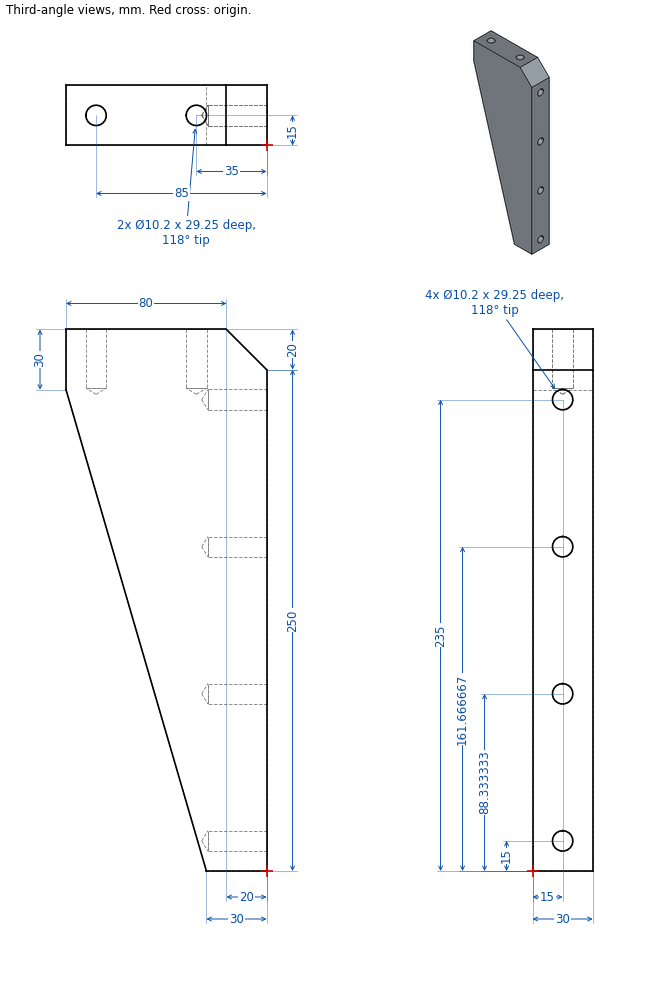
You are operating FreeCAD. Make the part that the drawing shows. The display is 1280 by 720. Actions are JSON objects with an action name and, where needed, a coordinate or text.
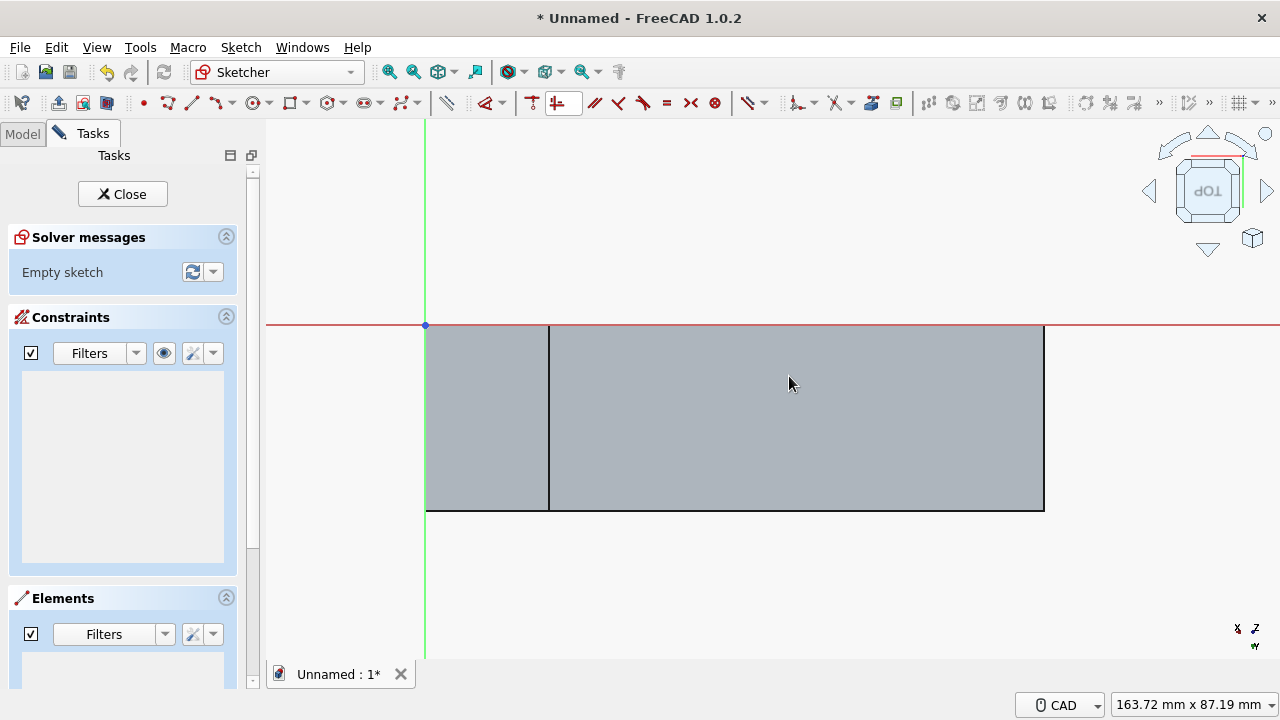
{"action": "key", "text": "g c"}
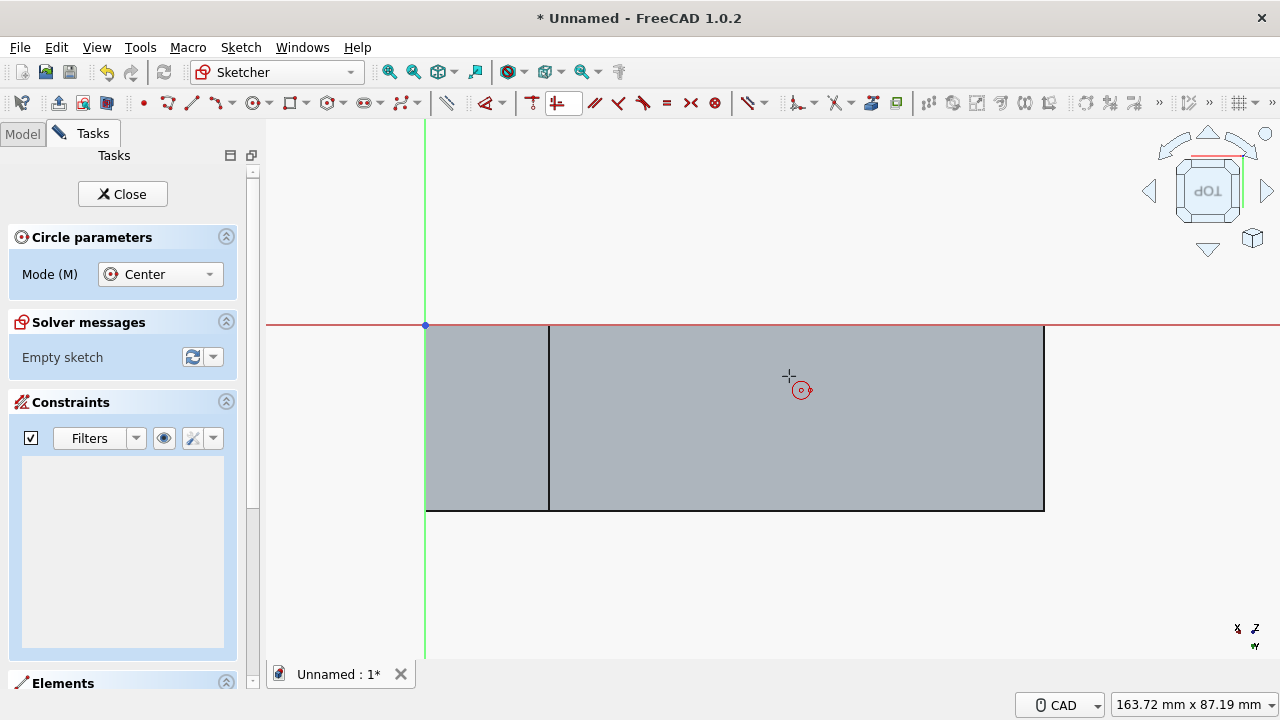
{"action": "left_click", "coordinate": [642, 418]}
{"action": "left_click", "coordinate": [664, 396]}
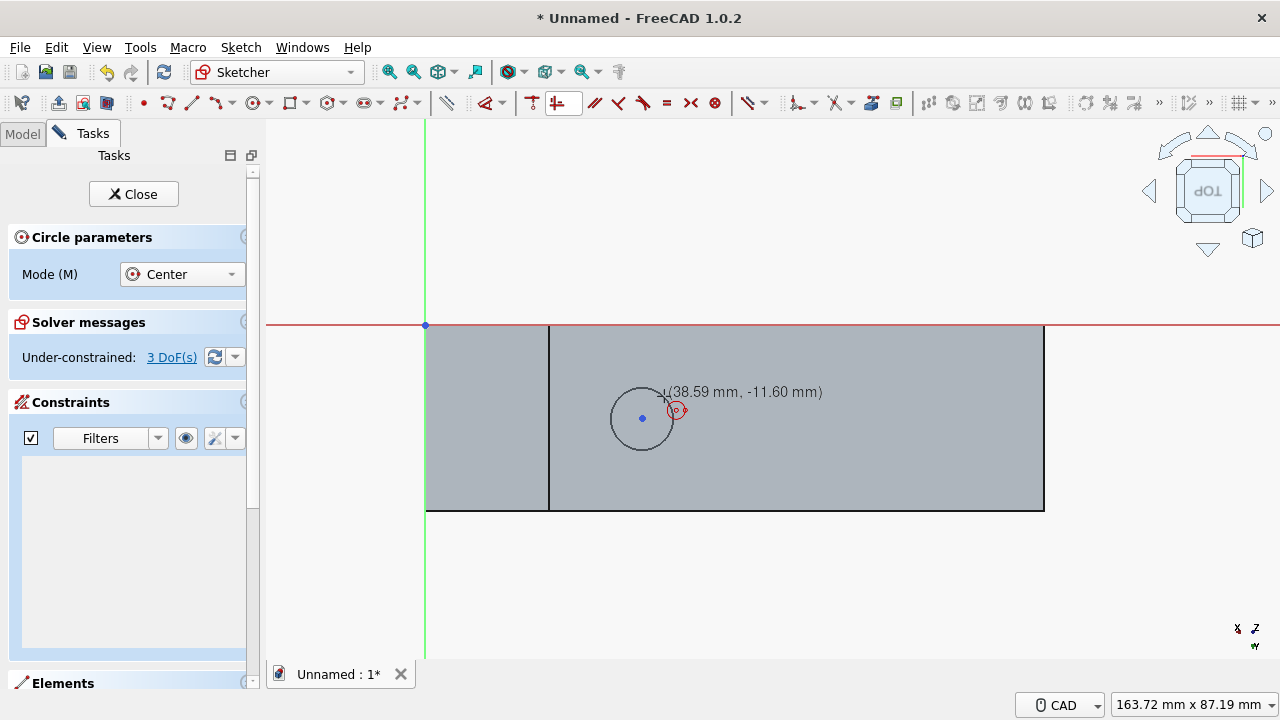
{"action": "left_click", "coordinate": [951, 418]}
{"action": "left_click", "coordinate": [974, 396]}
{"action": "key", "text": "Escape"}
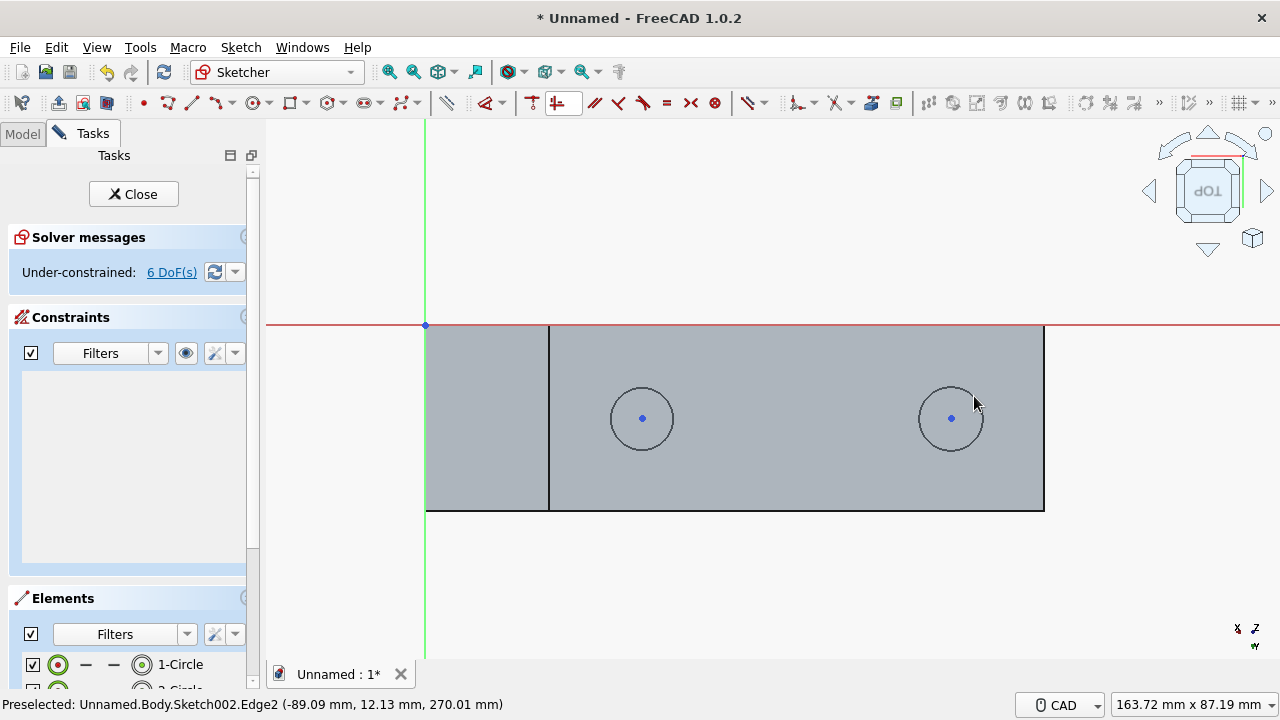
{"action": "left_click", "coordinate": [664, 397]}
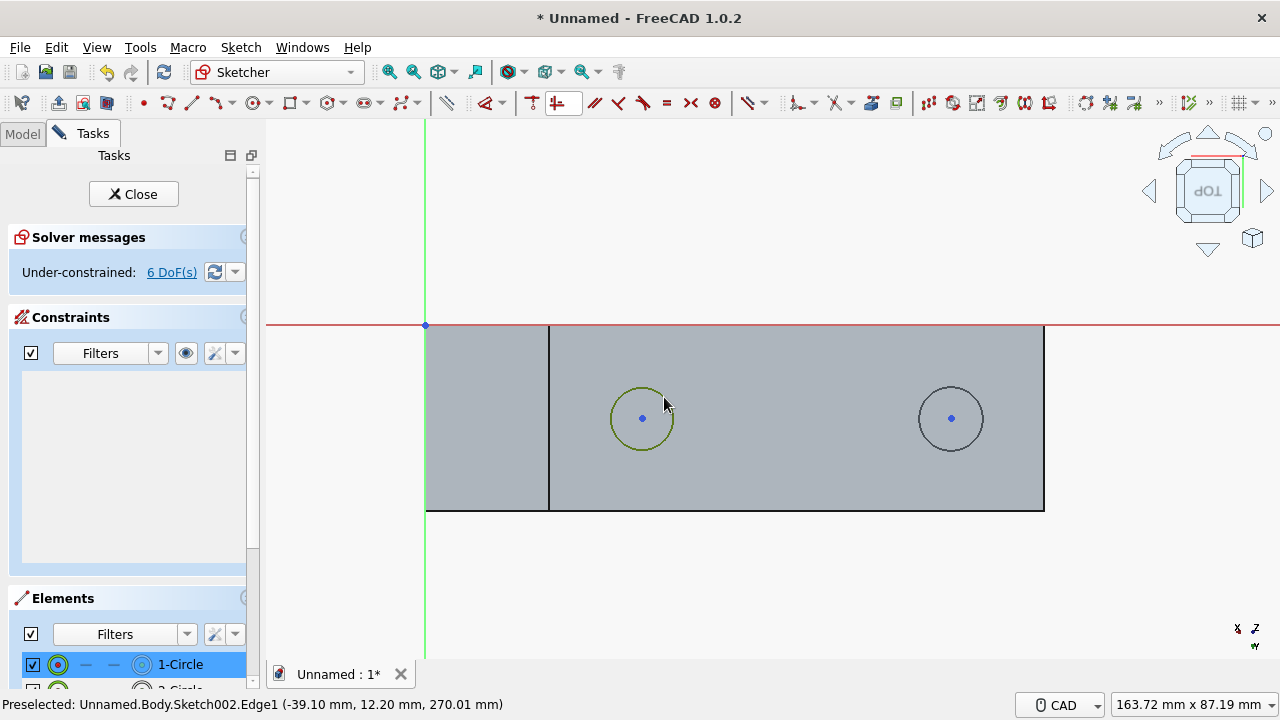
{"action": "left_click", "coordinate": [973, 396]}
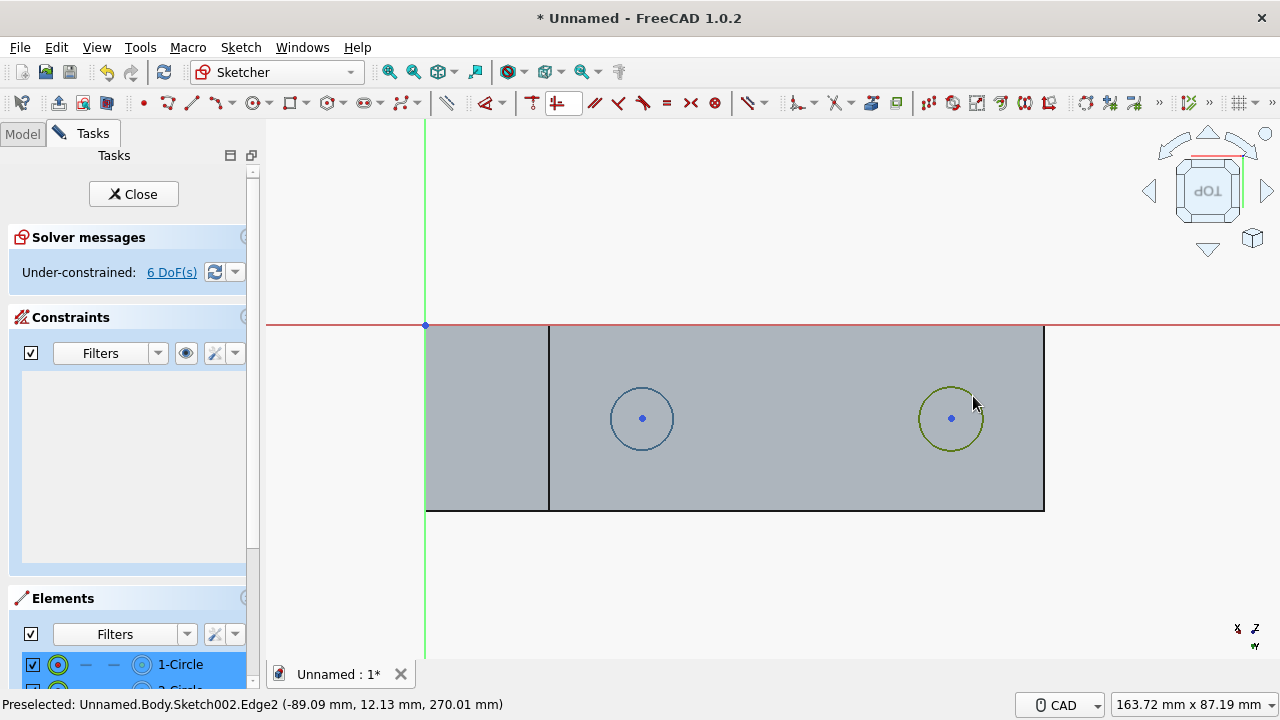
{"action": "key", "text": "e"}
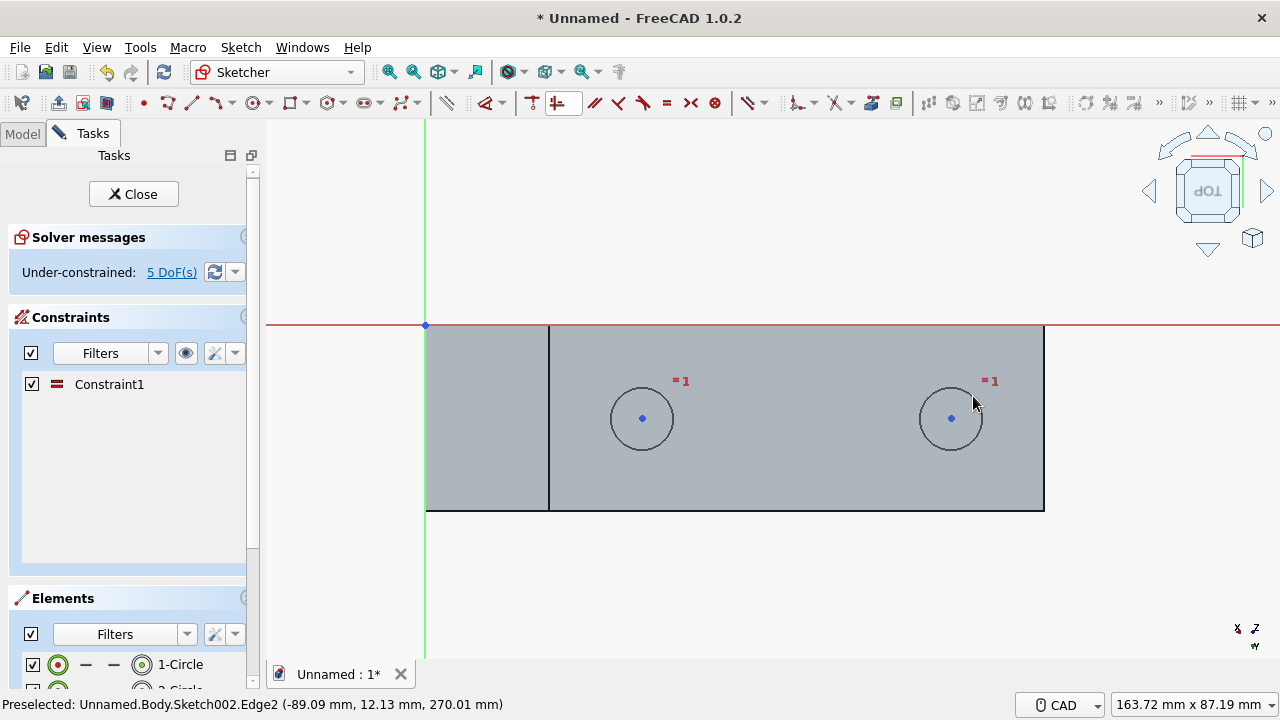
{"action": "left_click", "coordinate": [486, 104]}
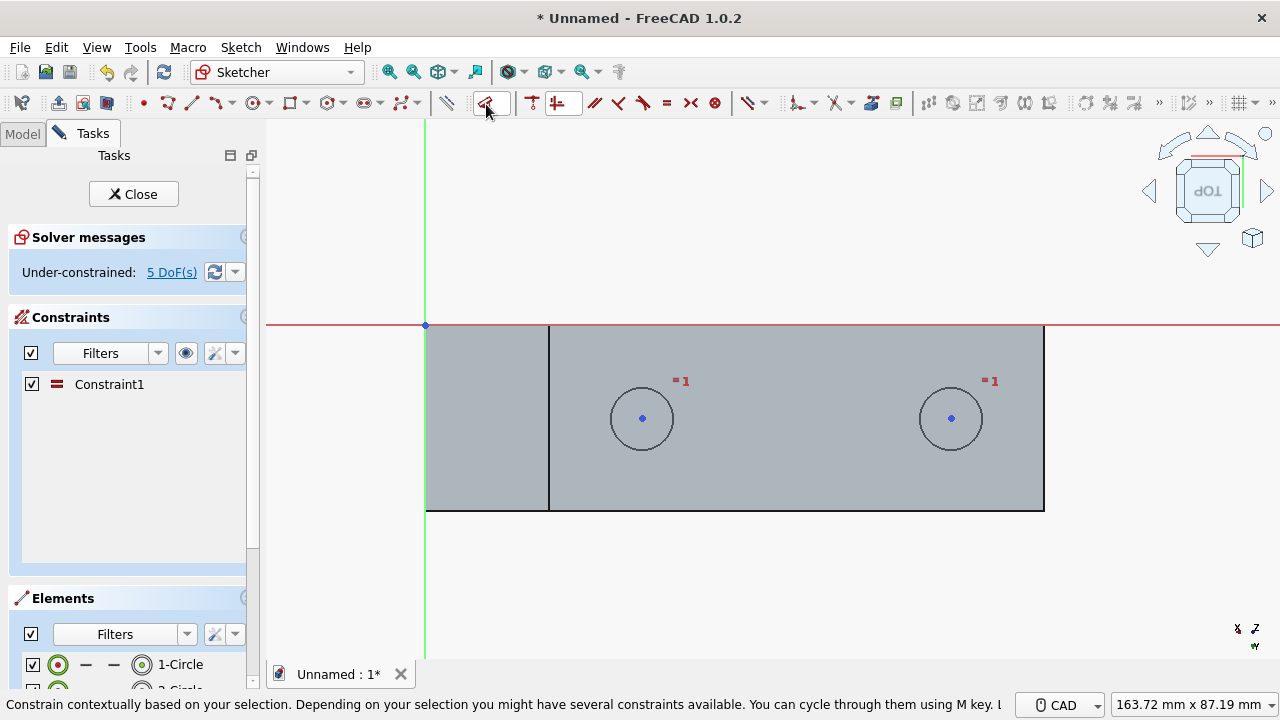
{"action": "left_click", "coordinate": [664, 397]}
{"action": "left_click", "coordinate": [687, 374]}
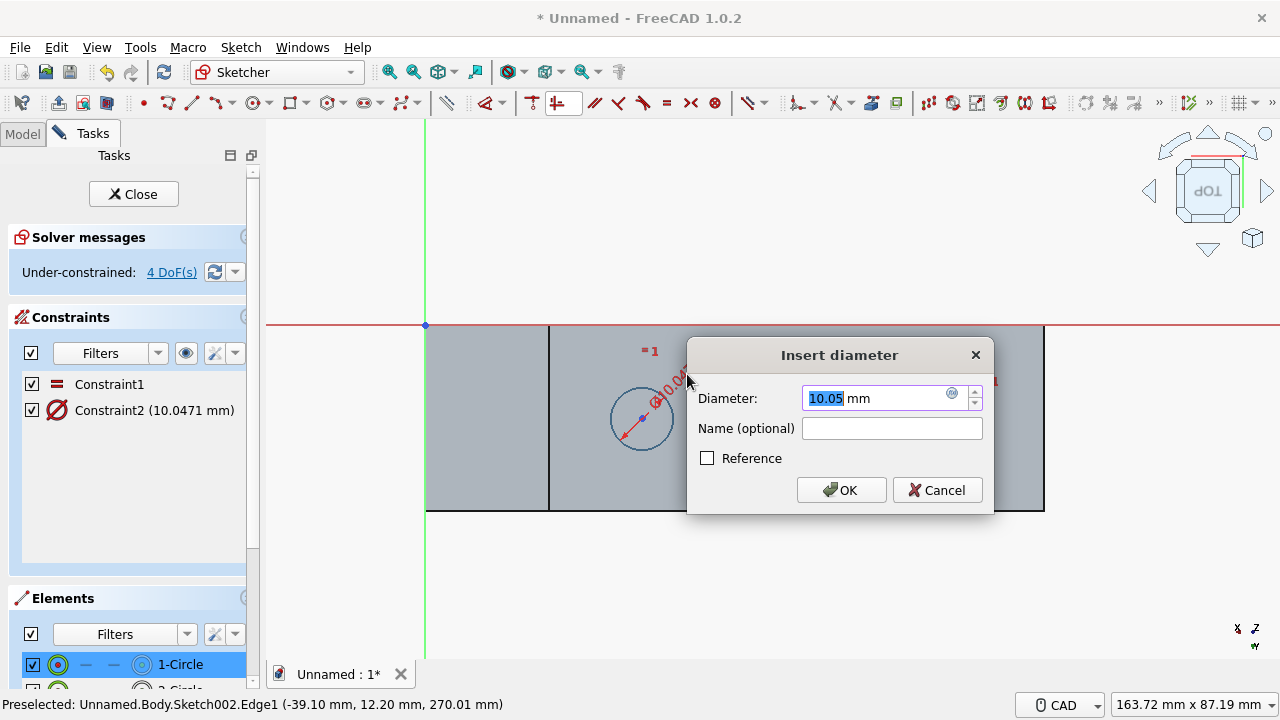
{"action": "type", "text": "10.2"}
{"action": "key", "text": "Return"}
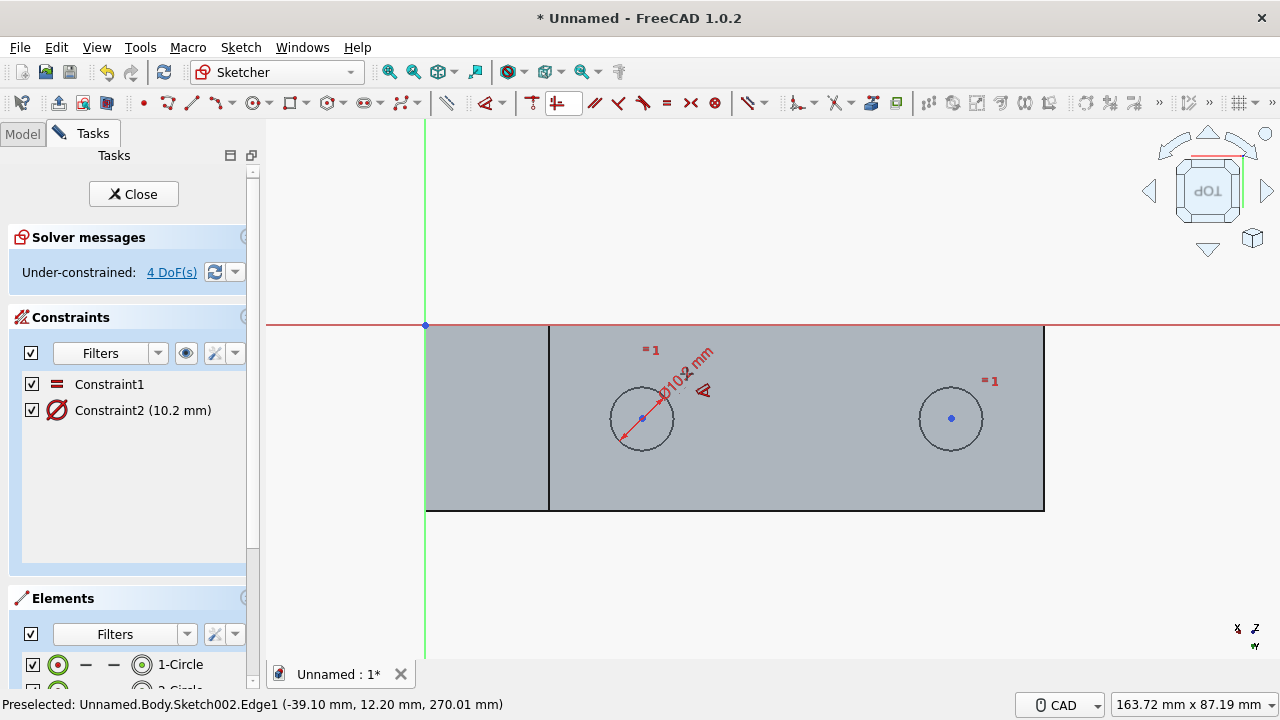
{"action": "left_click", "coordinate": [642, 419]}
{"action": "left_click", "coordinate": [534, 291]}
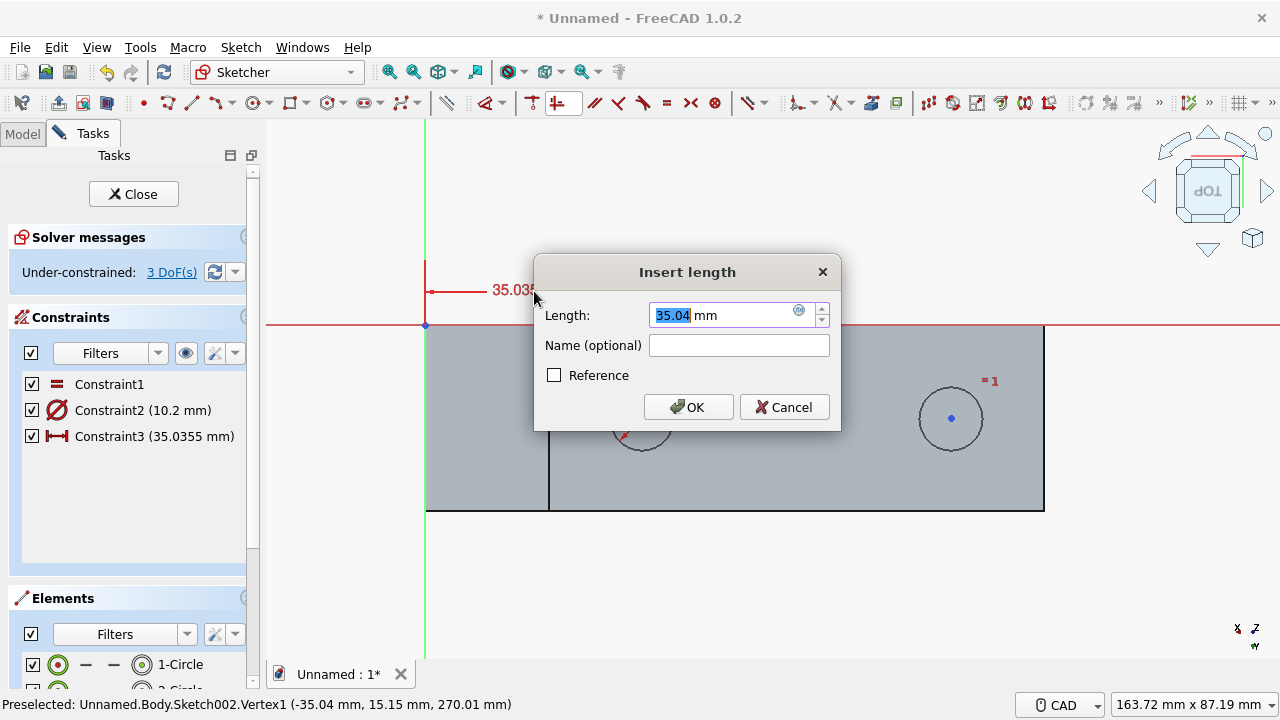
{"action": "type", "text": "35"}
{"action": "key", "text": "Return"}